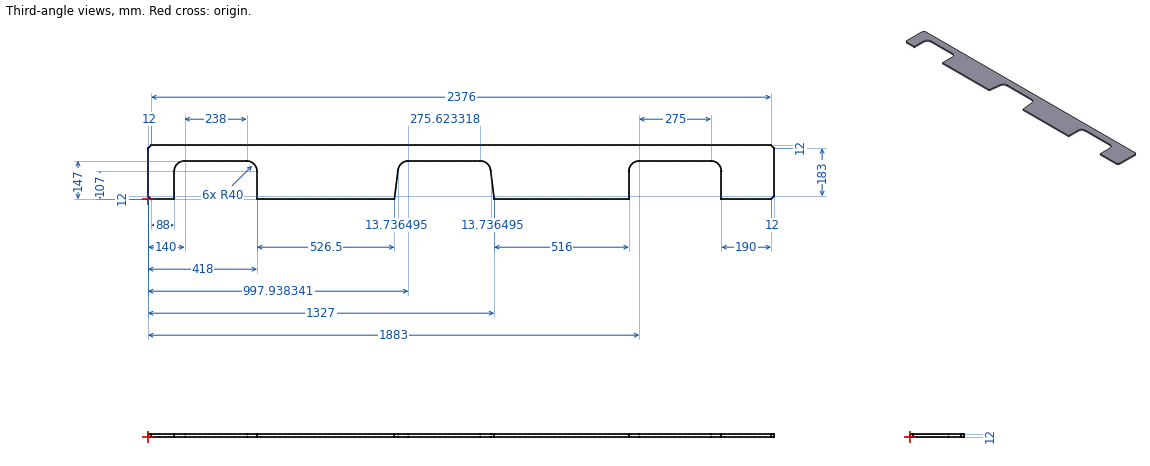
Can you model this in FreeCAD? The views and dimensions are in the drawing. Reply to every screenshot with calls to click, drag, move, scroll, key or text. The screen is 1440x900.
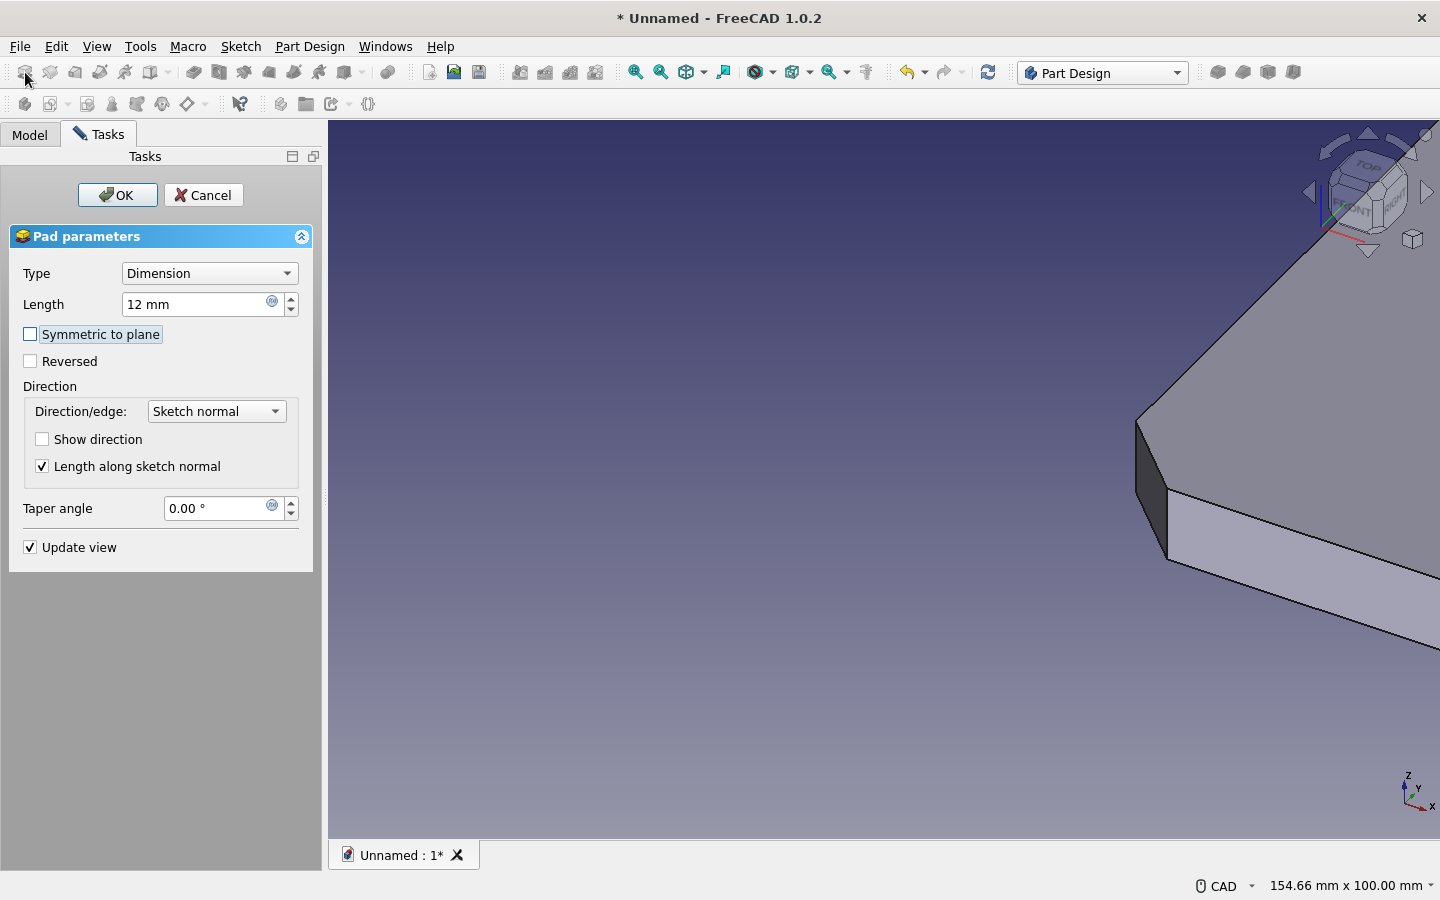
click(118, 195)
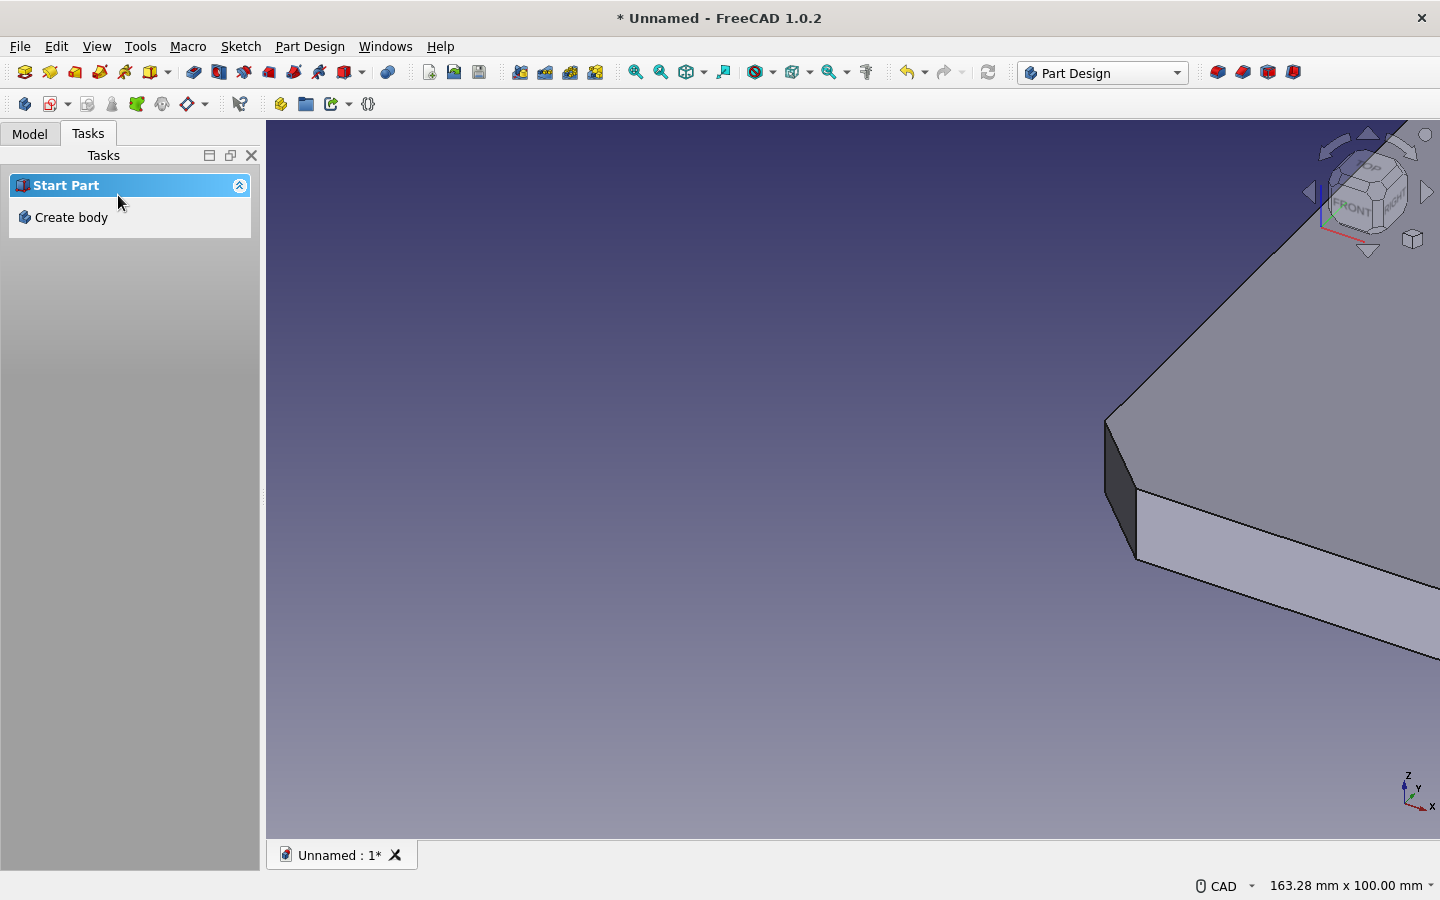
key(0)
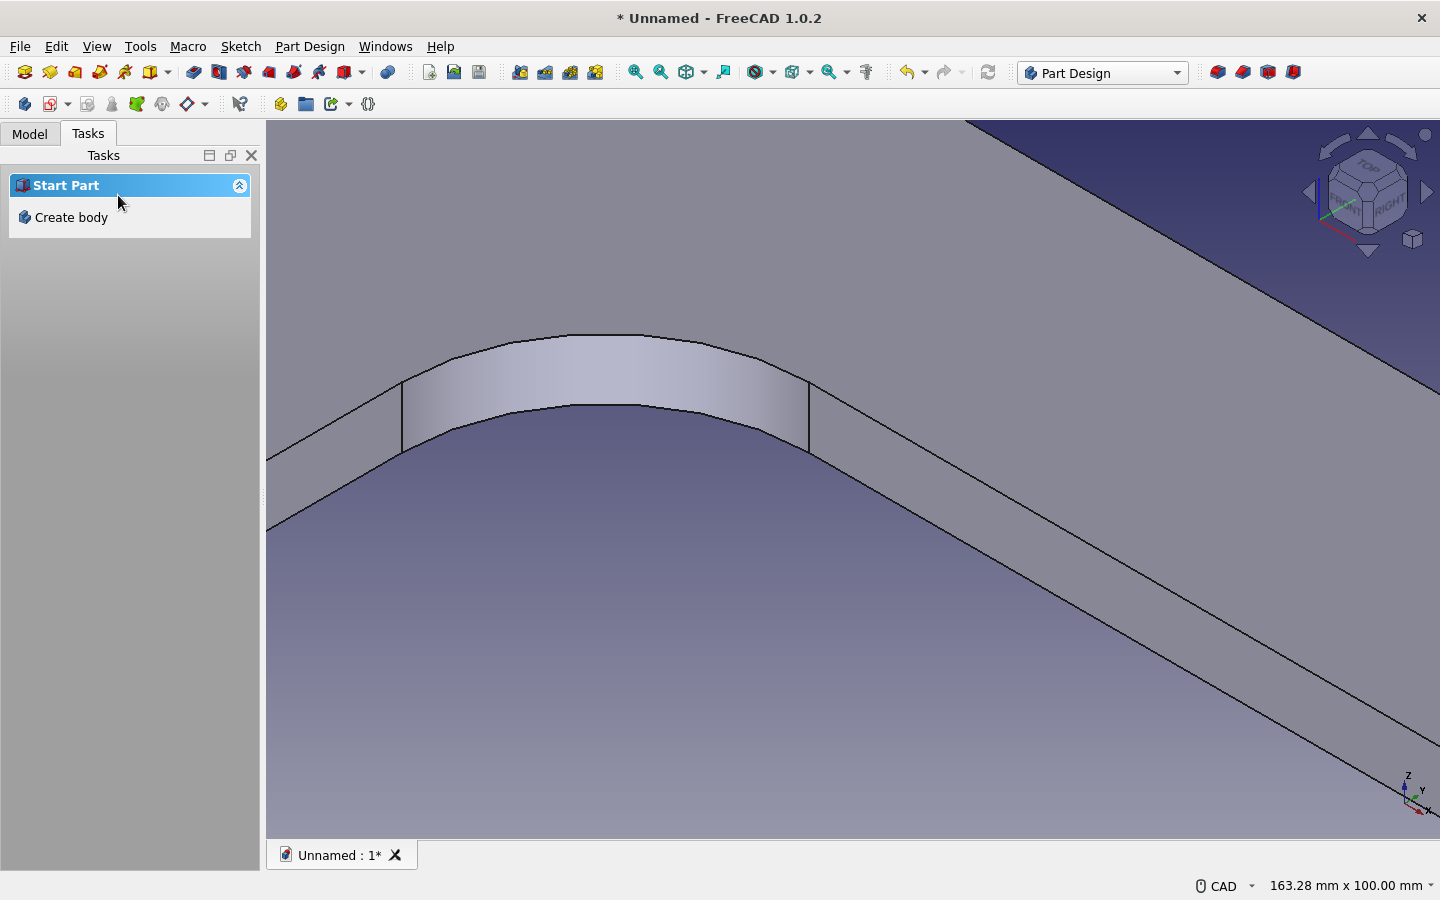
click(636, 72)